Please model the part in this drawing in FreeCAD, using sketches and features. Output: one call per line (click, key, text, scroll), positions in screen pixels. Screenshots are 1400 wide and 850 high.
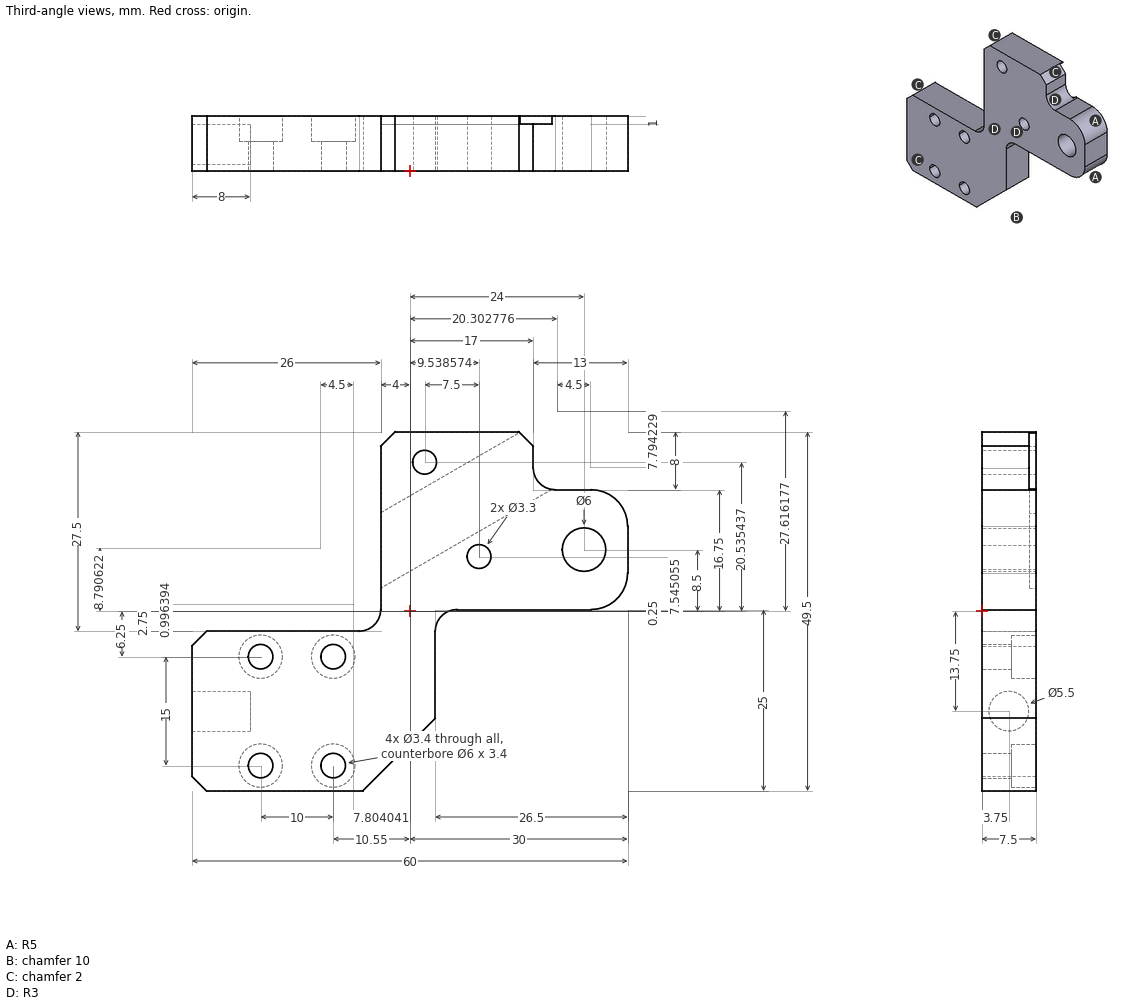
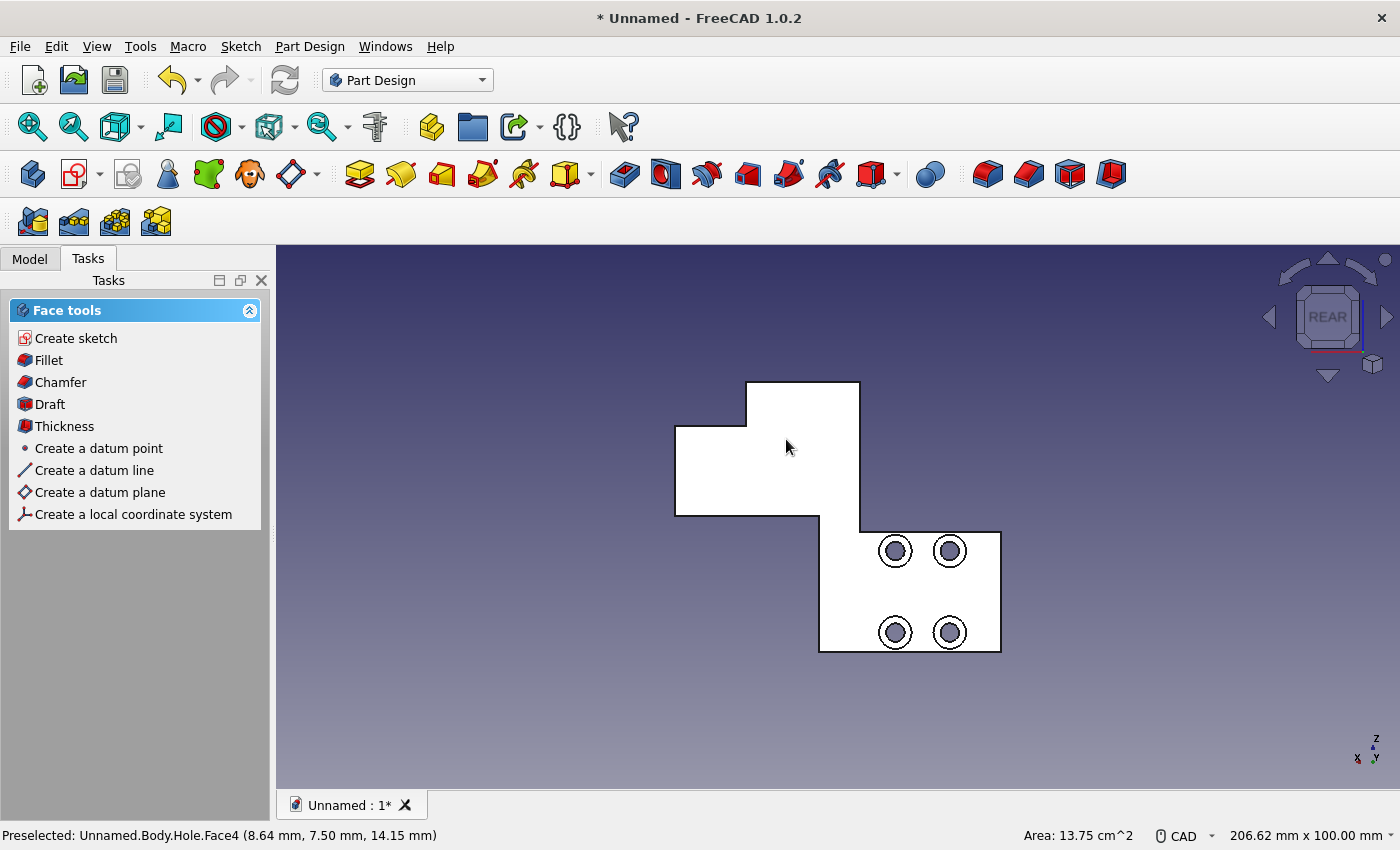
click(74, 174)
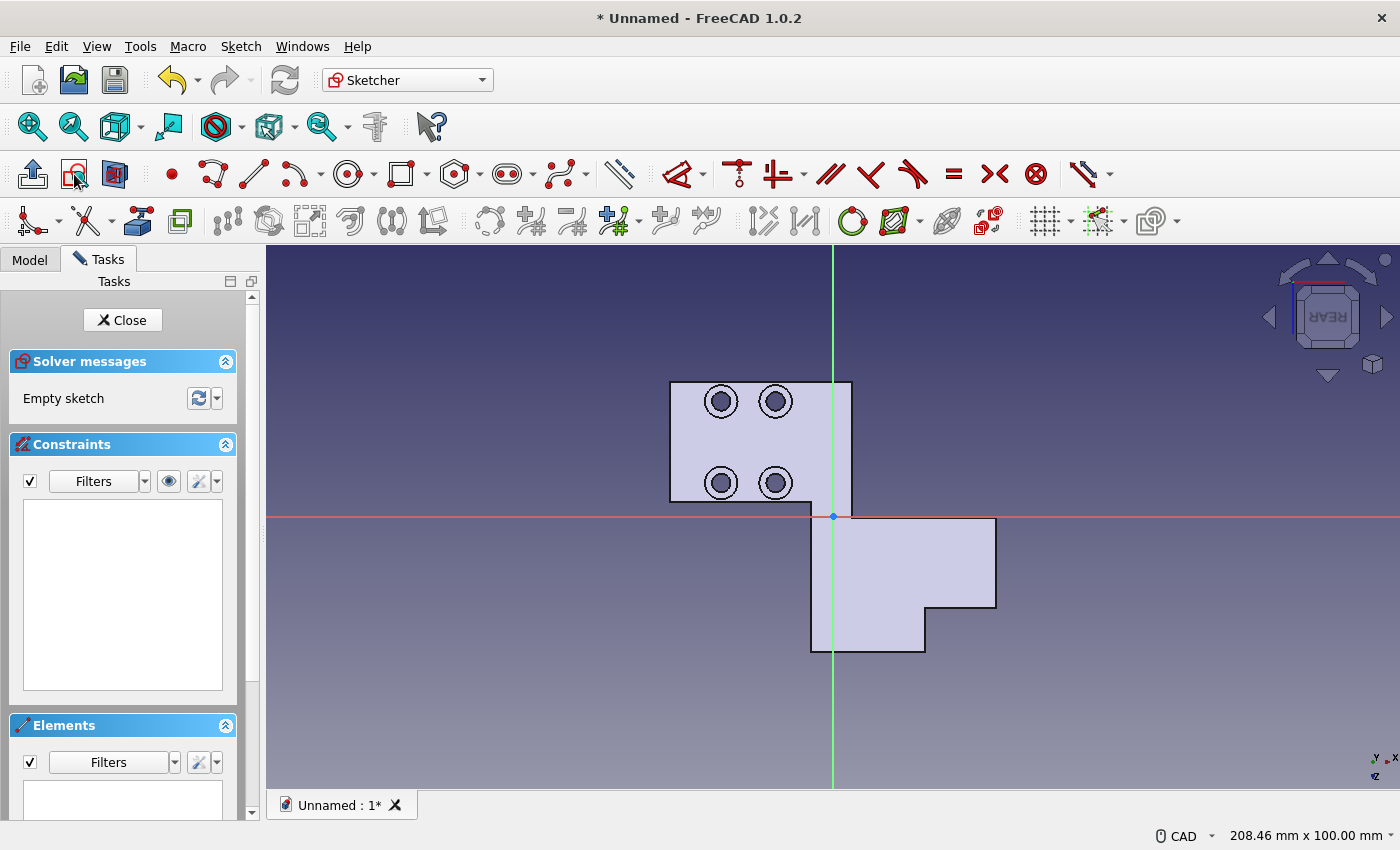
scroll(983, 568, up, 12)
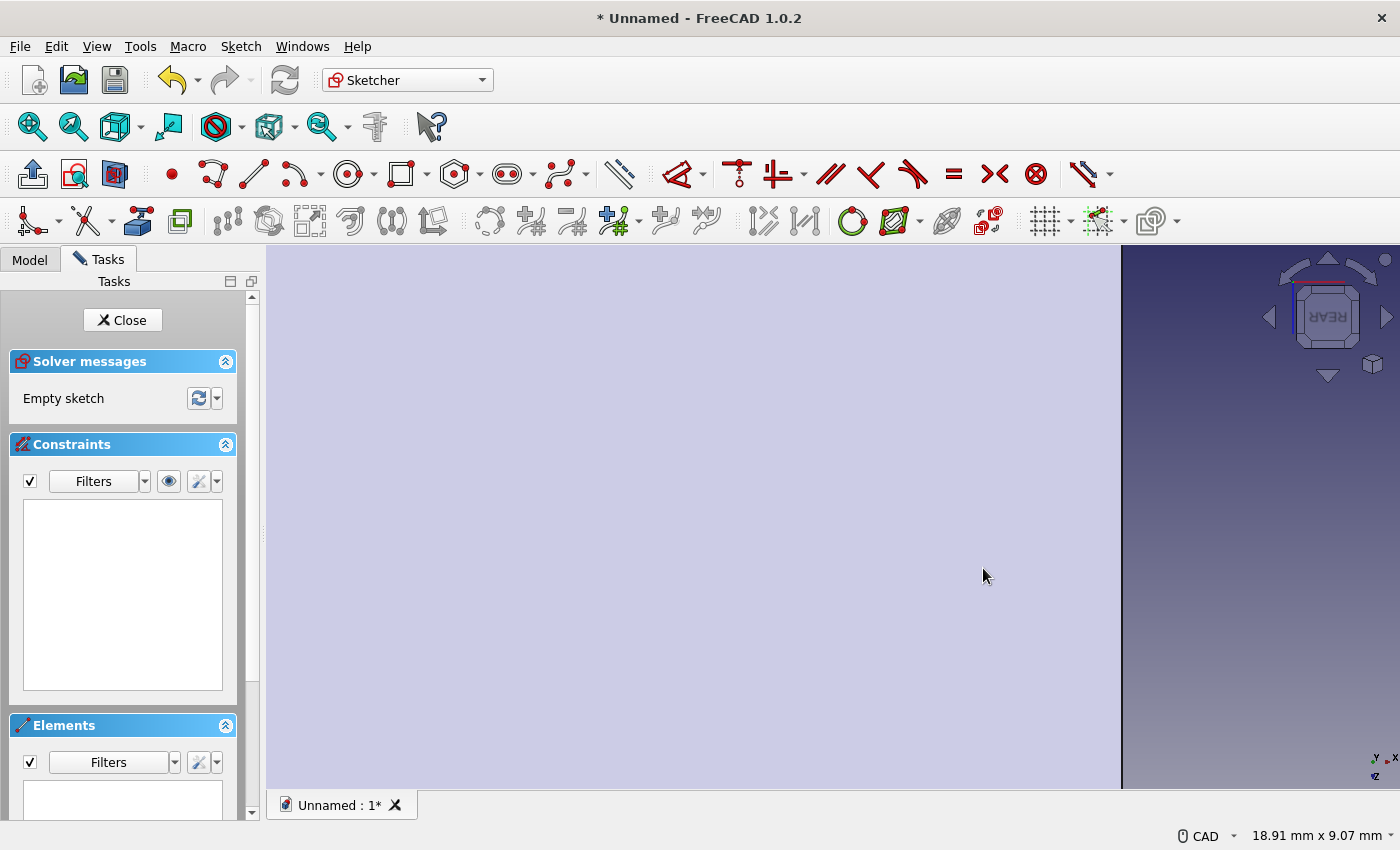
click(348, 174)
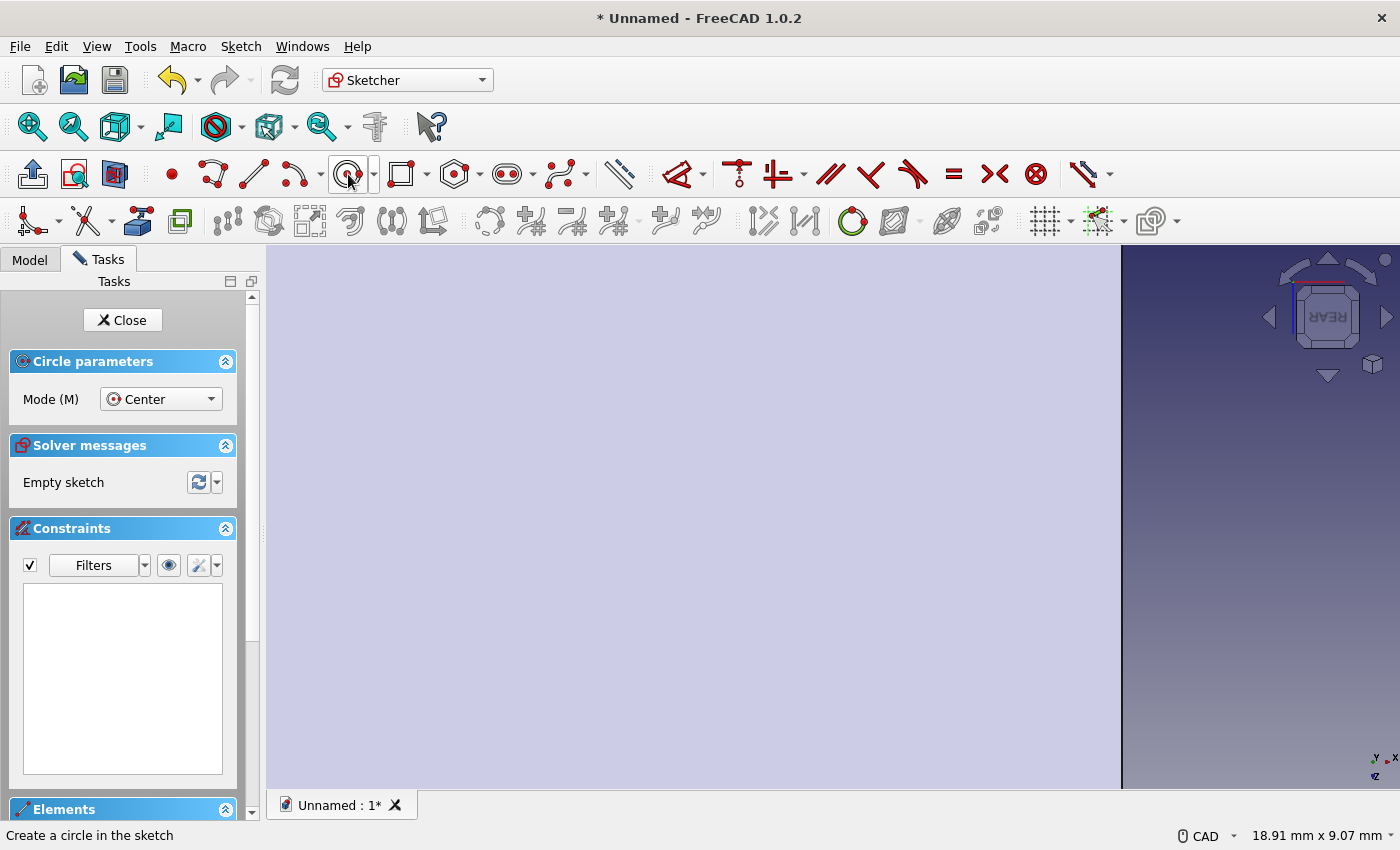
click(762, 510)
move(890, 382)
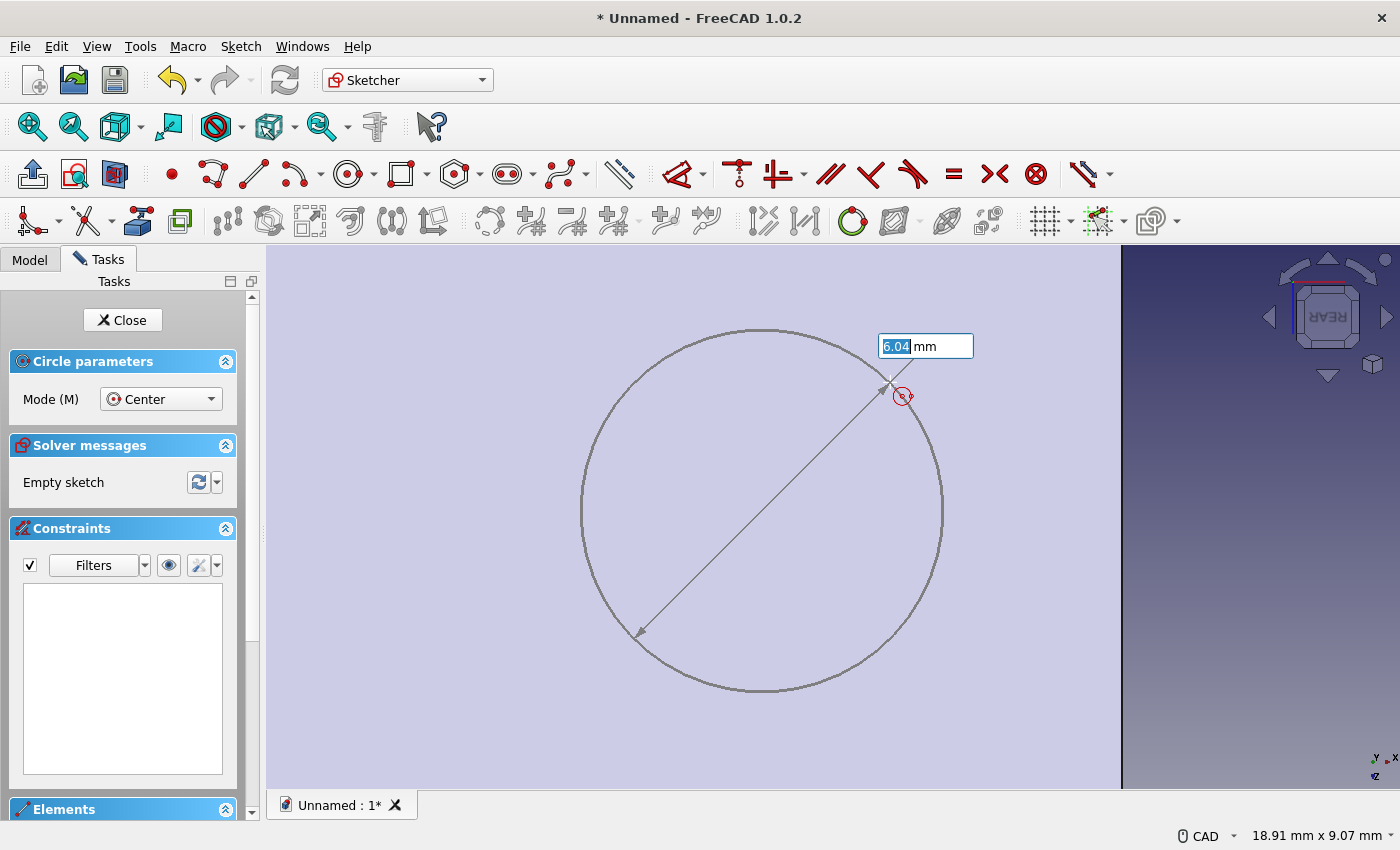
text(6)
key(Return)
key(Escape)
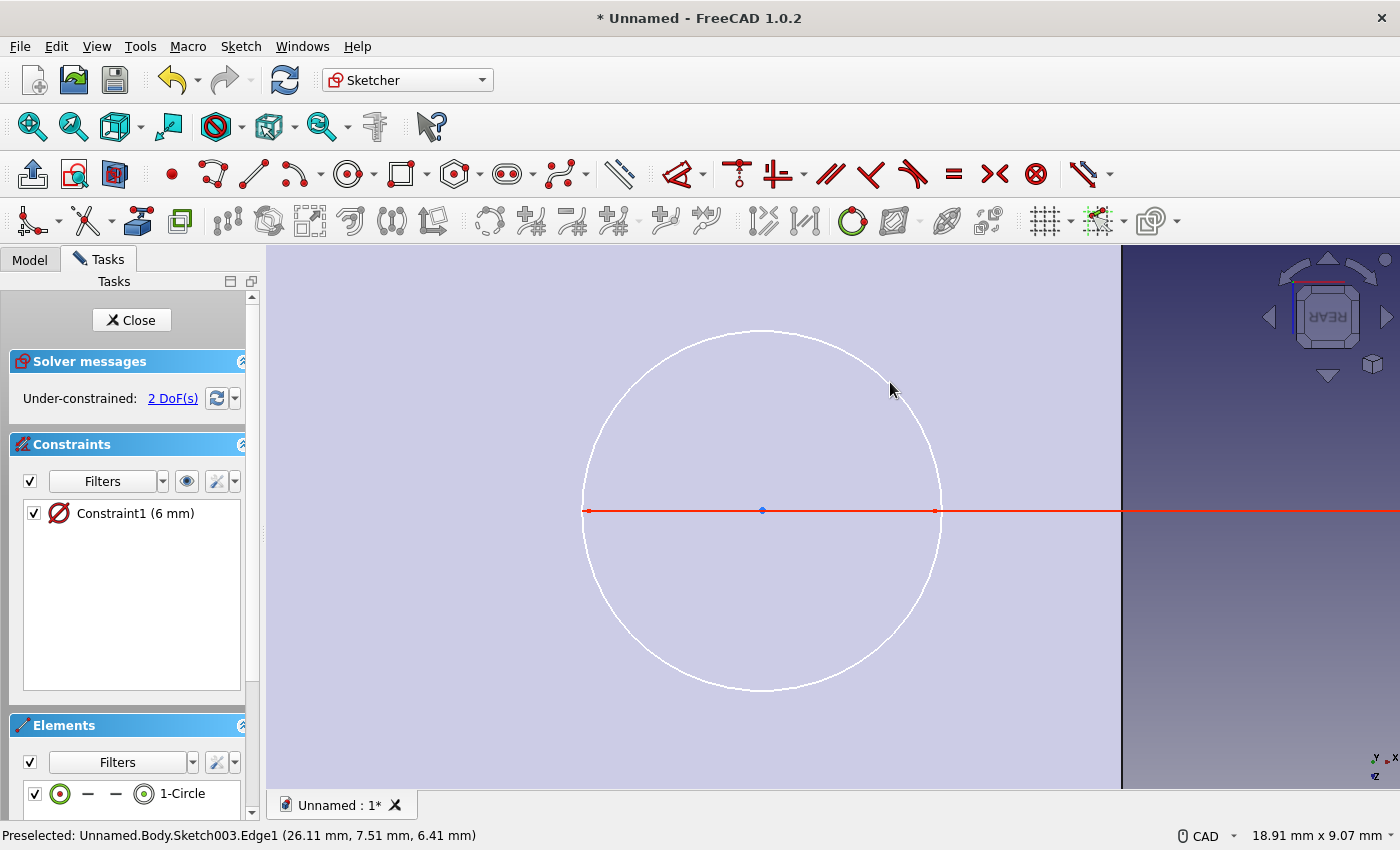
key(d)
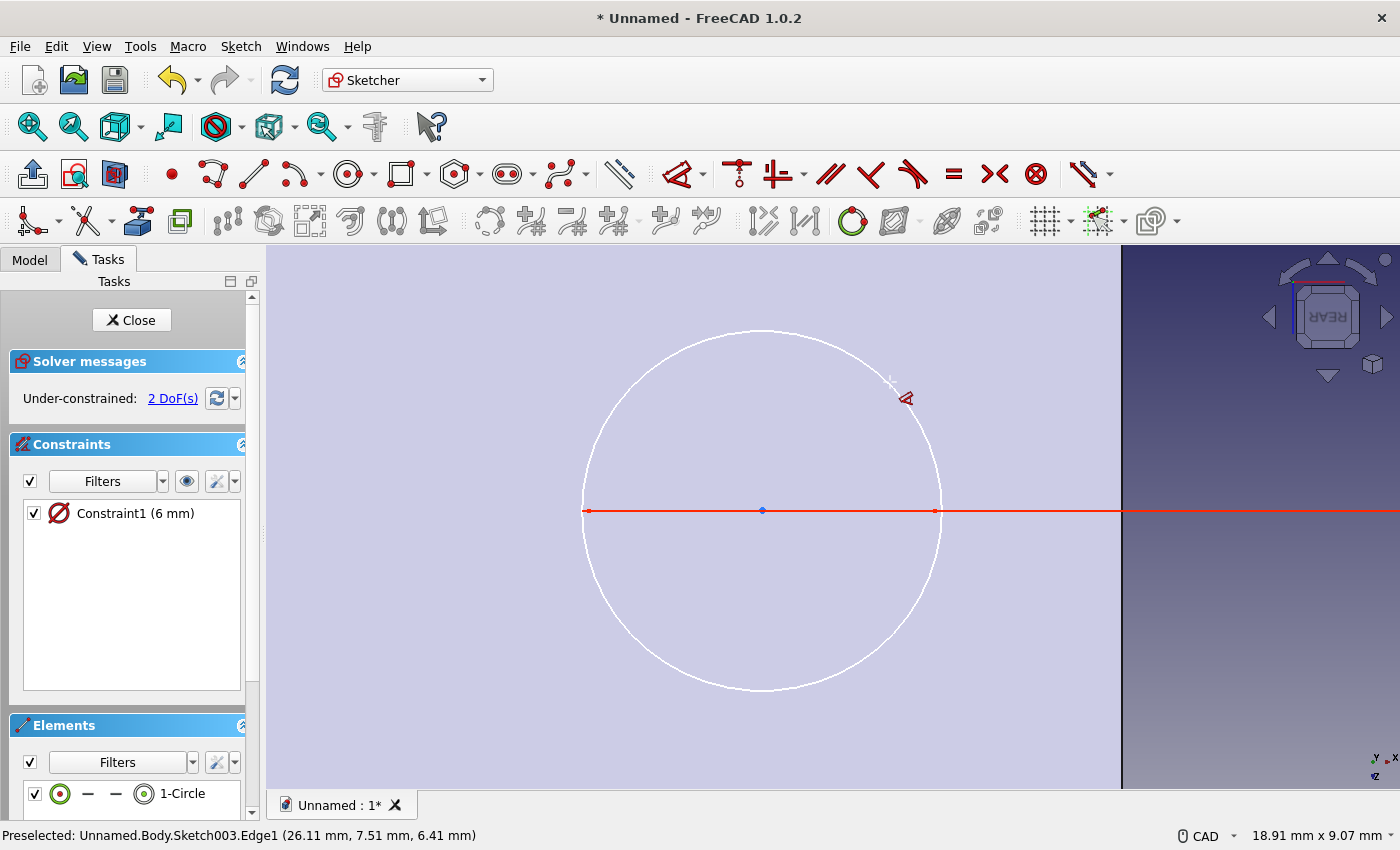
click(762, 511)
click(528, 545)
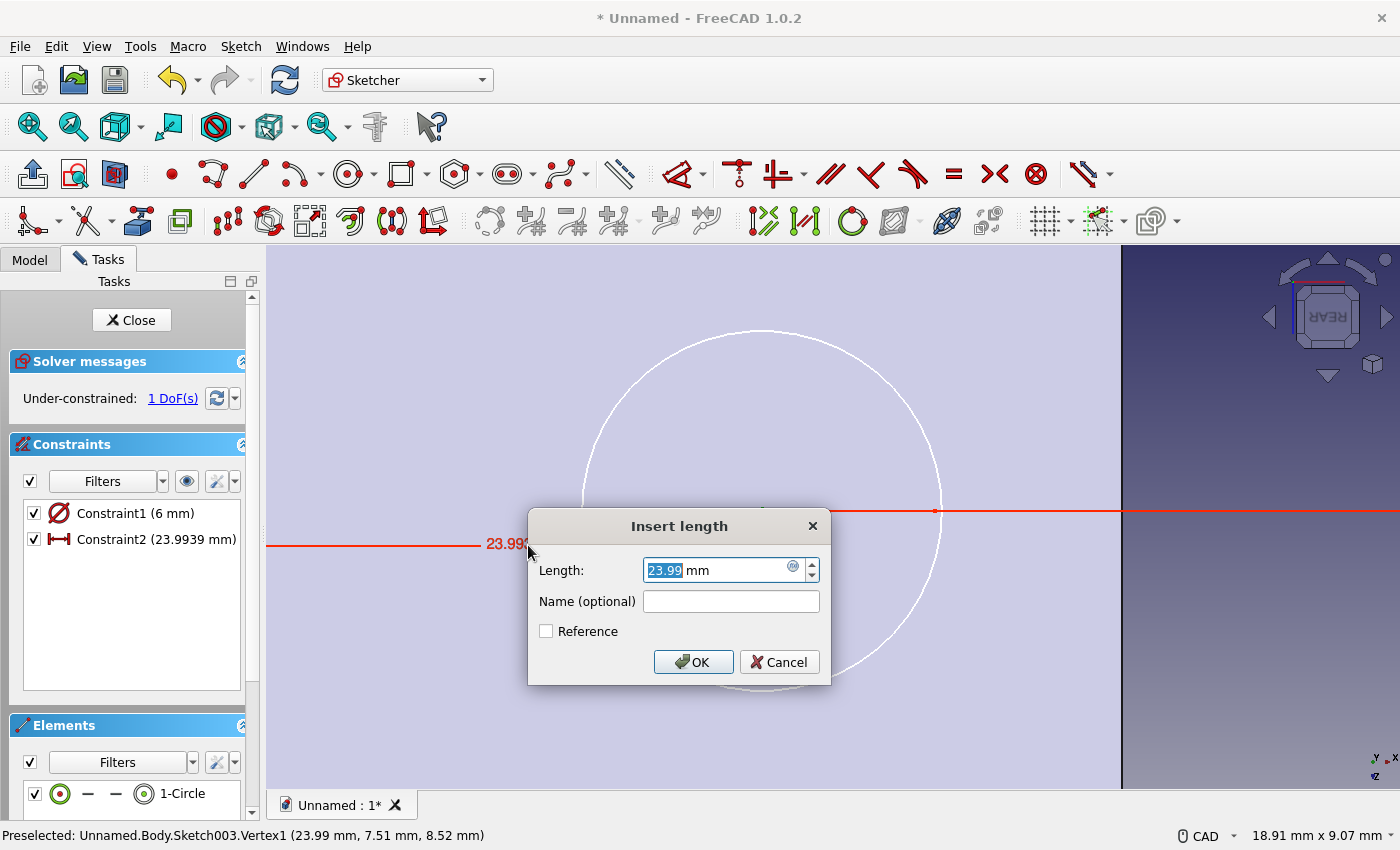
text(24)
key(Return)